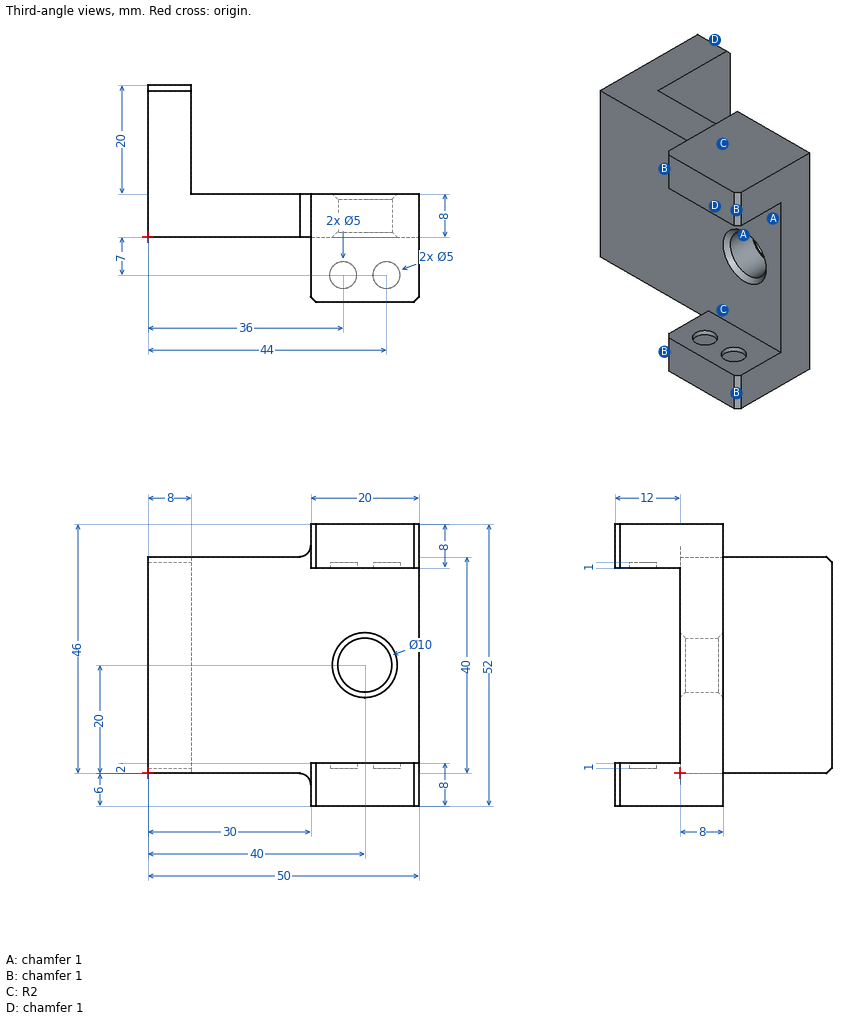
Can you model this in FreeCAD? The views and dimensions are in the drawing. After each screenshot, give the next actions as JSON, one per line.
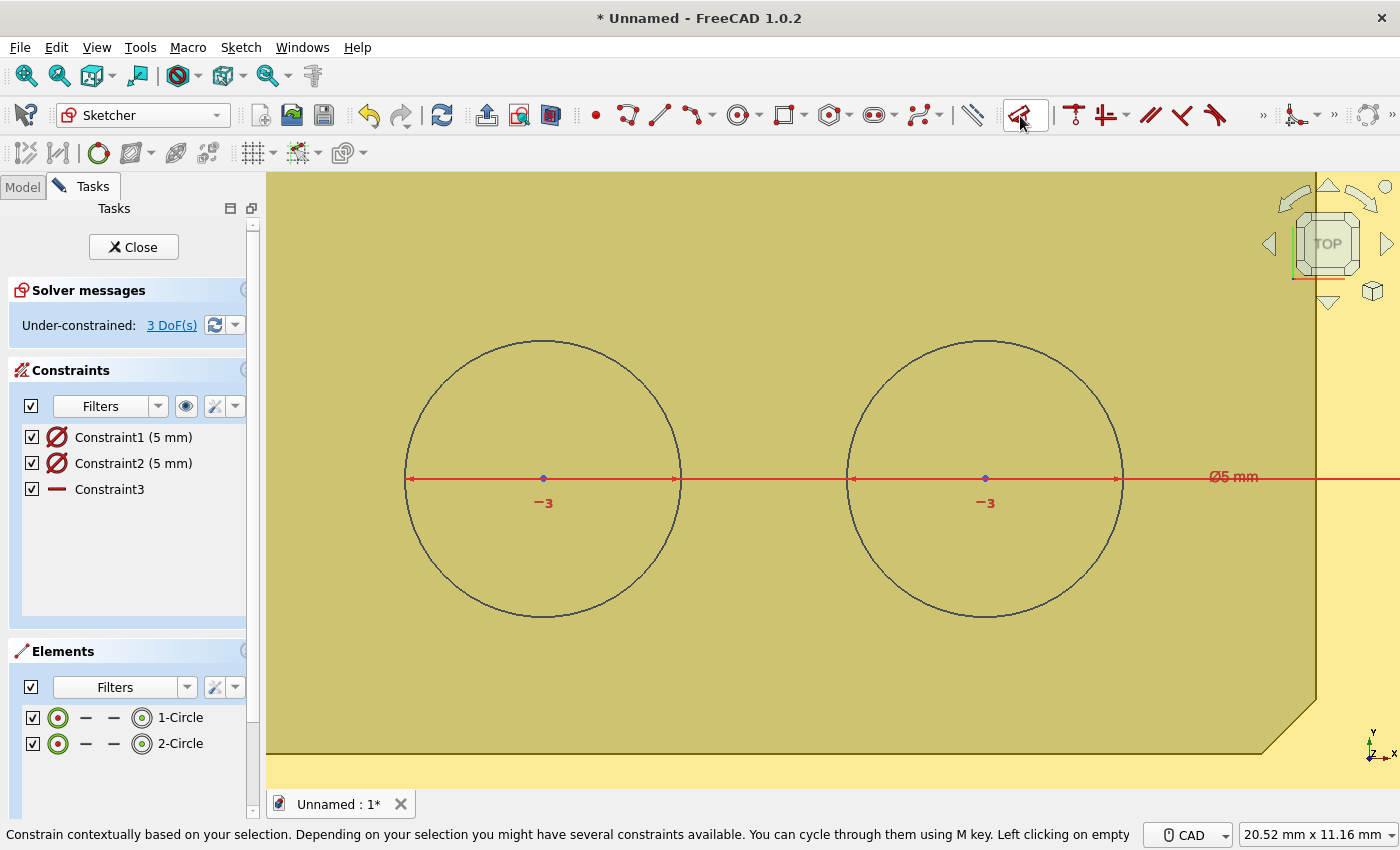
{"action": "left_click", "coordinate": [985, 479]}
{"action": "left_click", "coordinate": [1019, 275]}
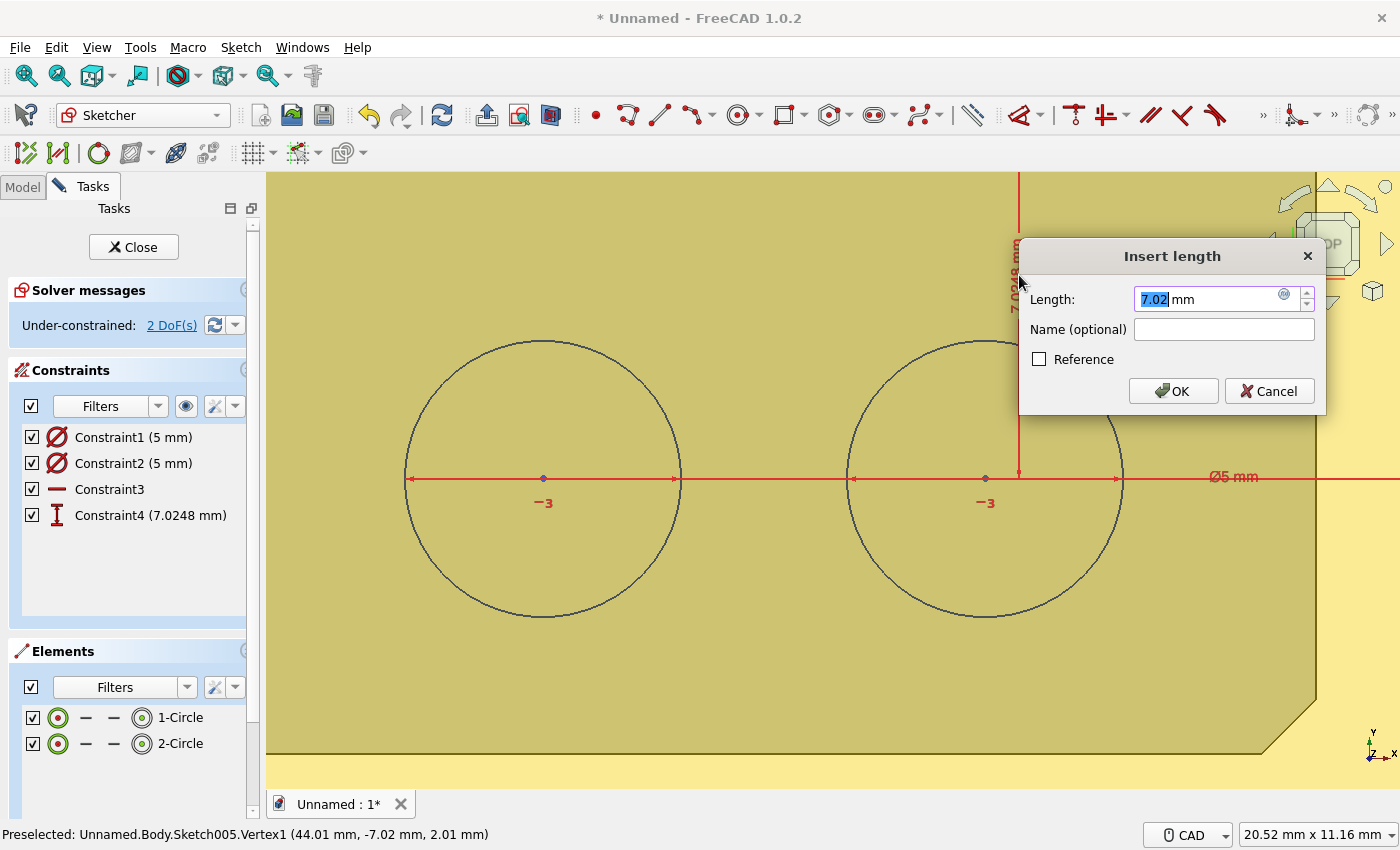
{"action": "type", "text": "7"}
{"action": "key", "text": "Return"}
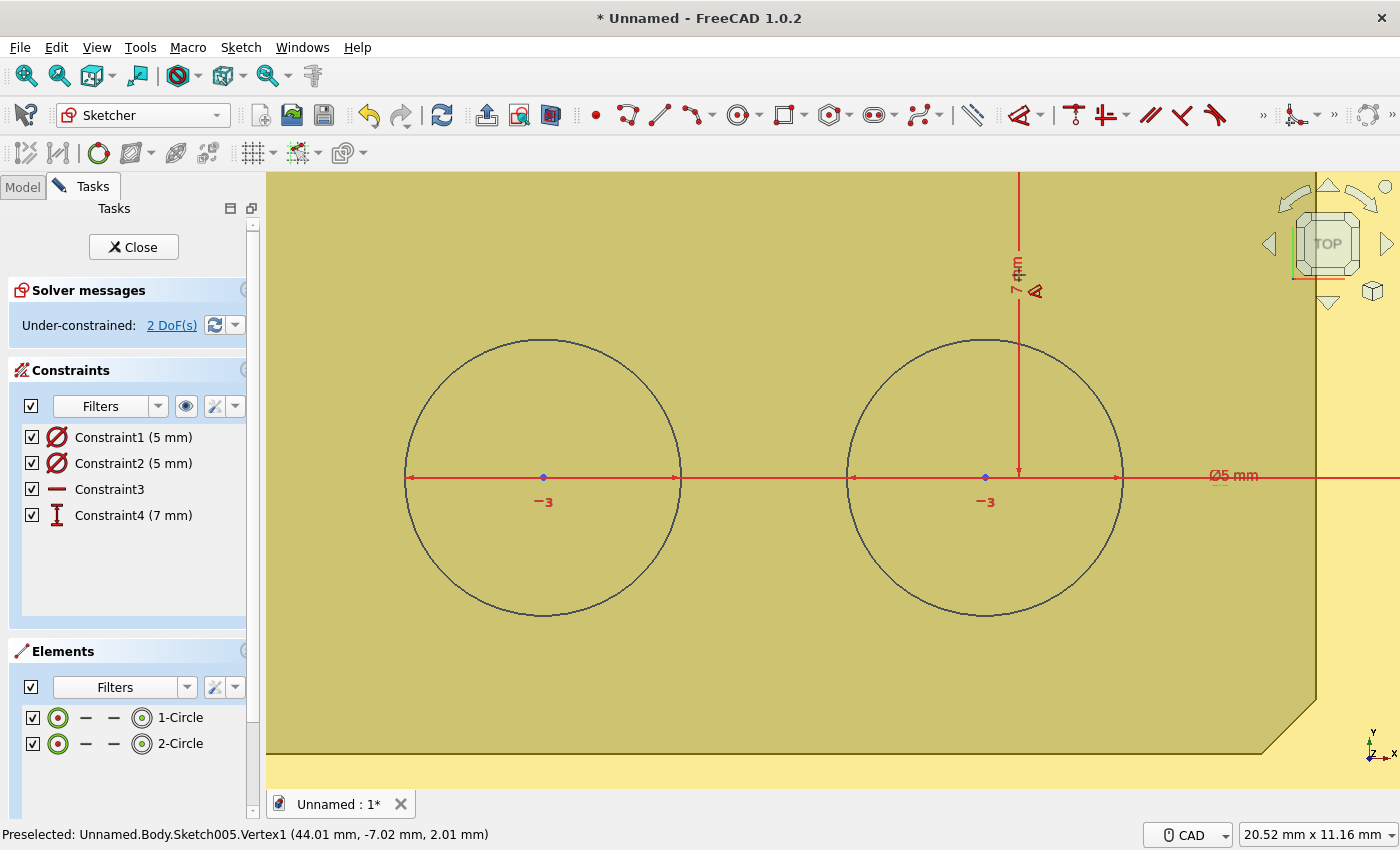
{"action": "left_click", "coordinate": [985, 478]}
{"action": "left_click", "coordinate": [640, 512]}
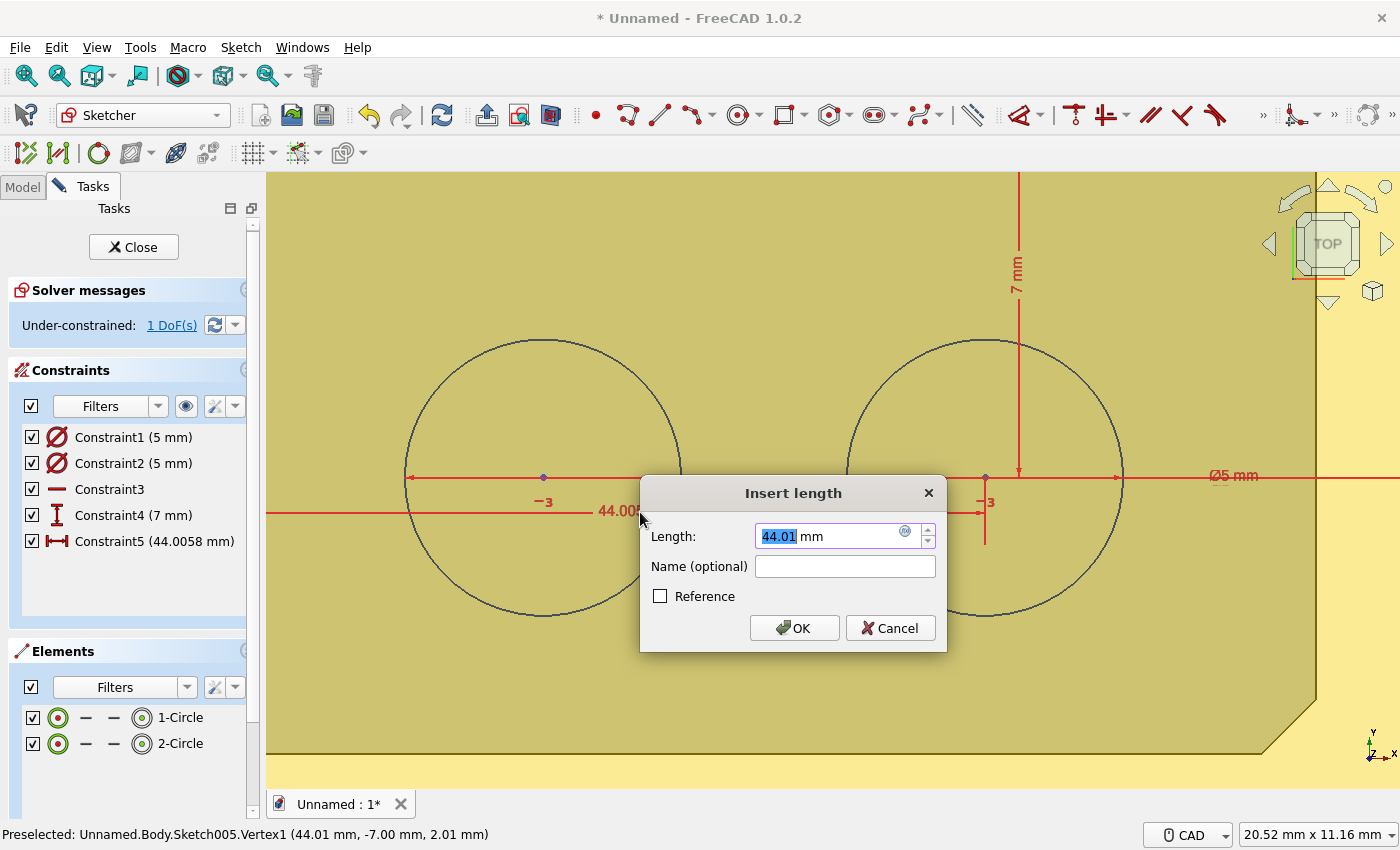
{"action": "type", "text": "44"}
{"action": "key", "text": "Return"}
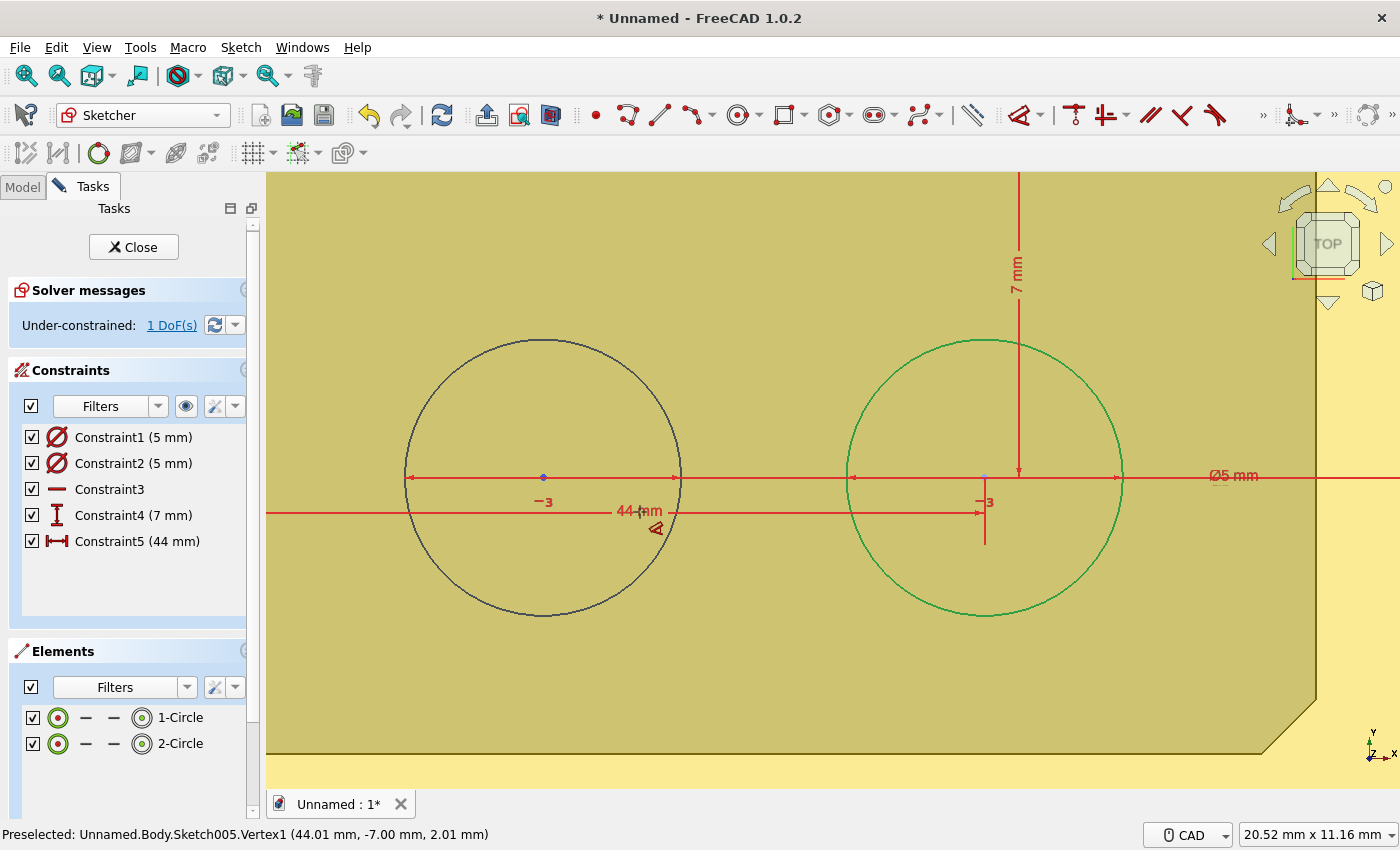
{"action": "left_click", "coordinate": [543, 478]}
{"action": "left_click", "coordinate": [361, 512]}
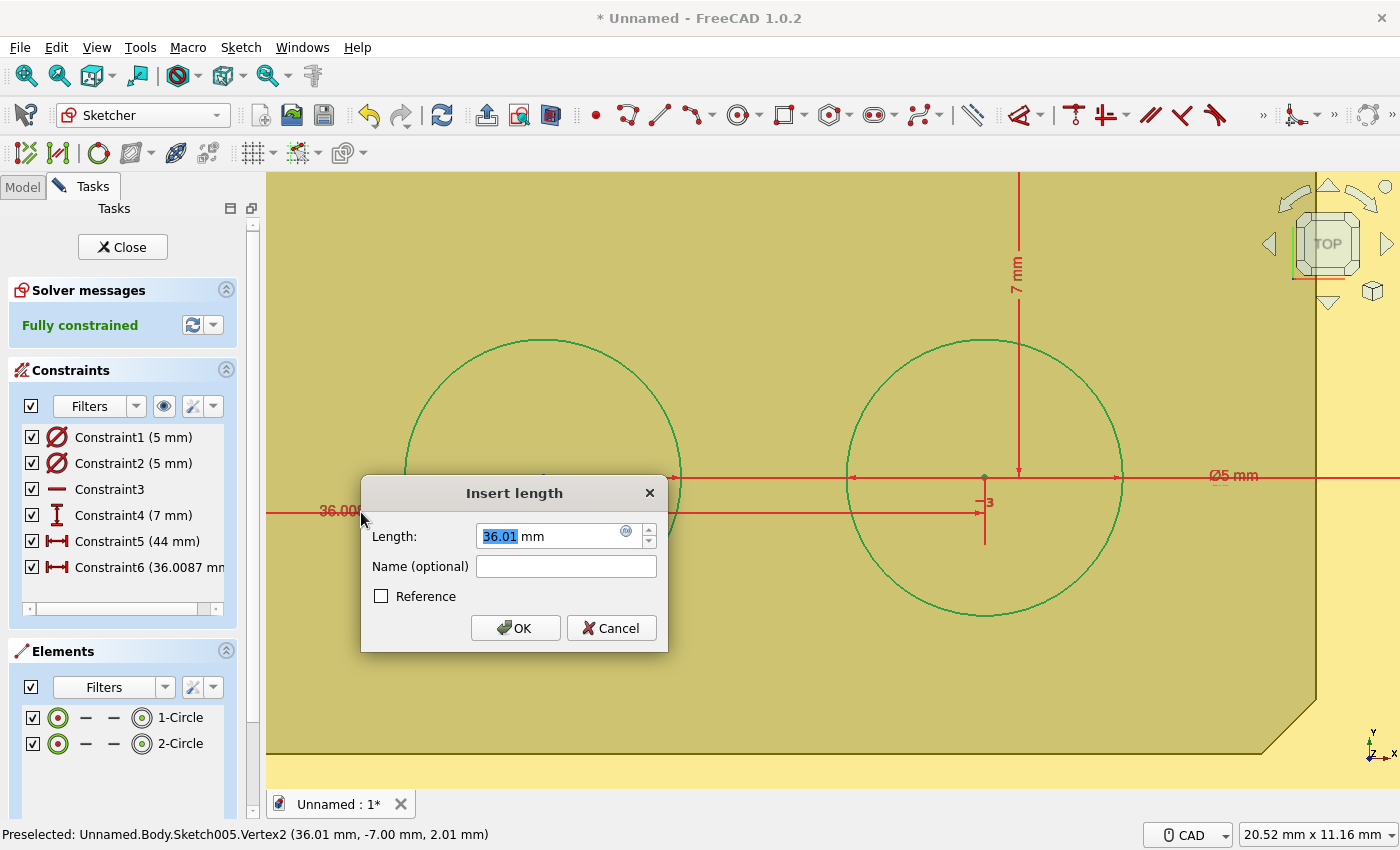
{"action": "type", "text": "36"}
{"action": "key", "text": "Return"}
{"action": "key", "text": "Escape"}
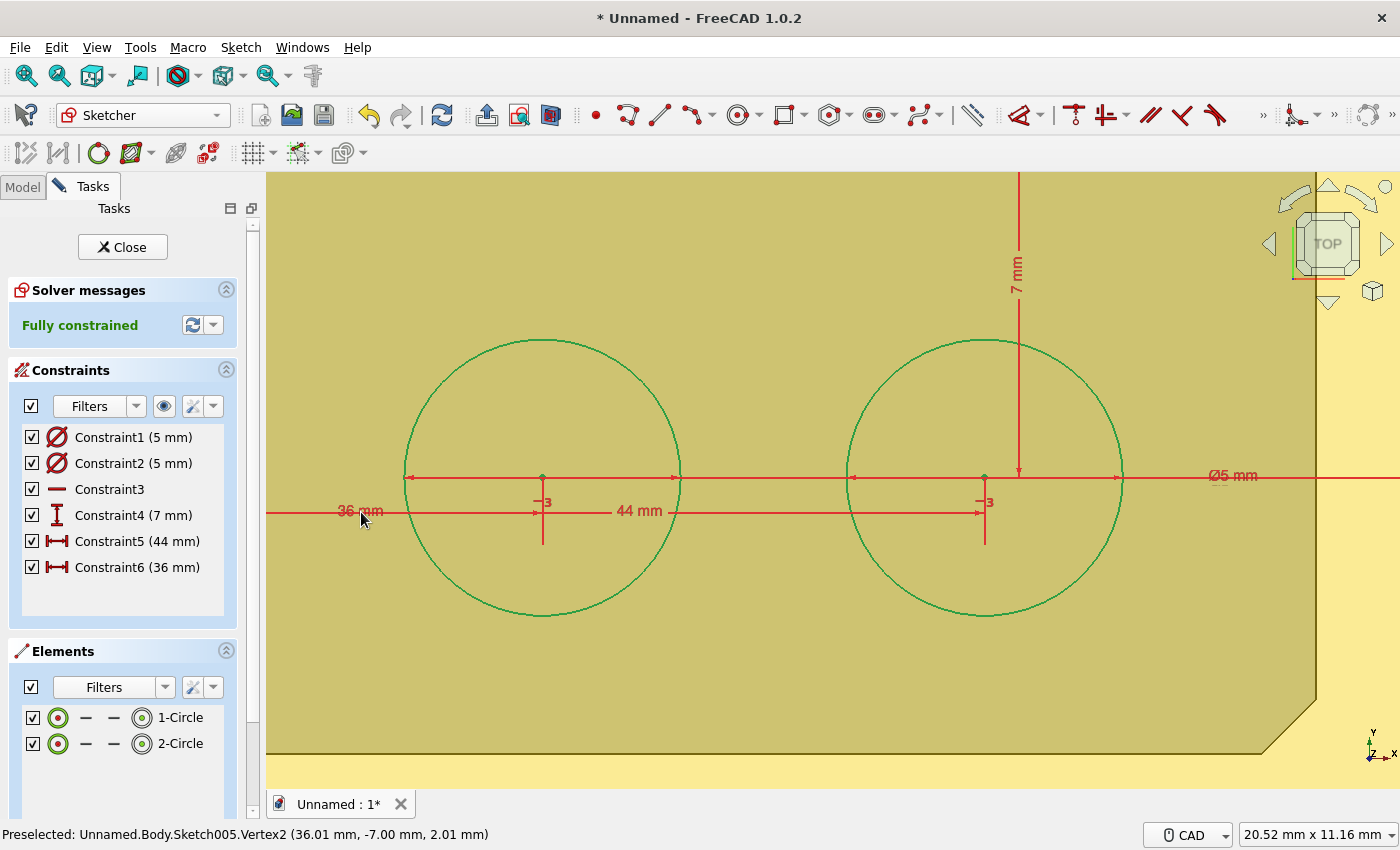
{"action": "left_click", "coordinate": [123, 247]}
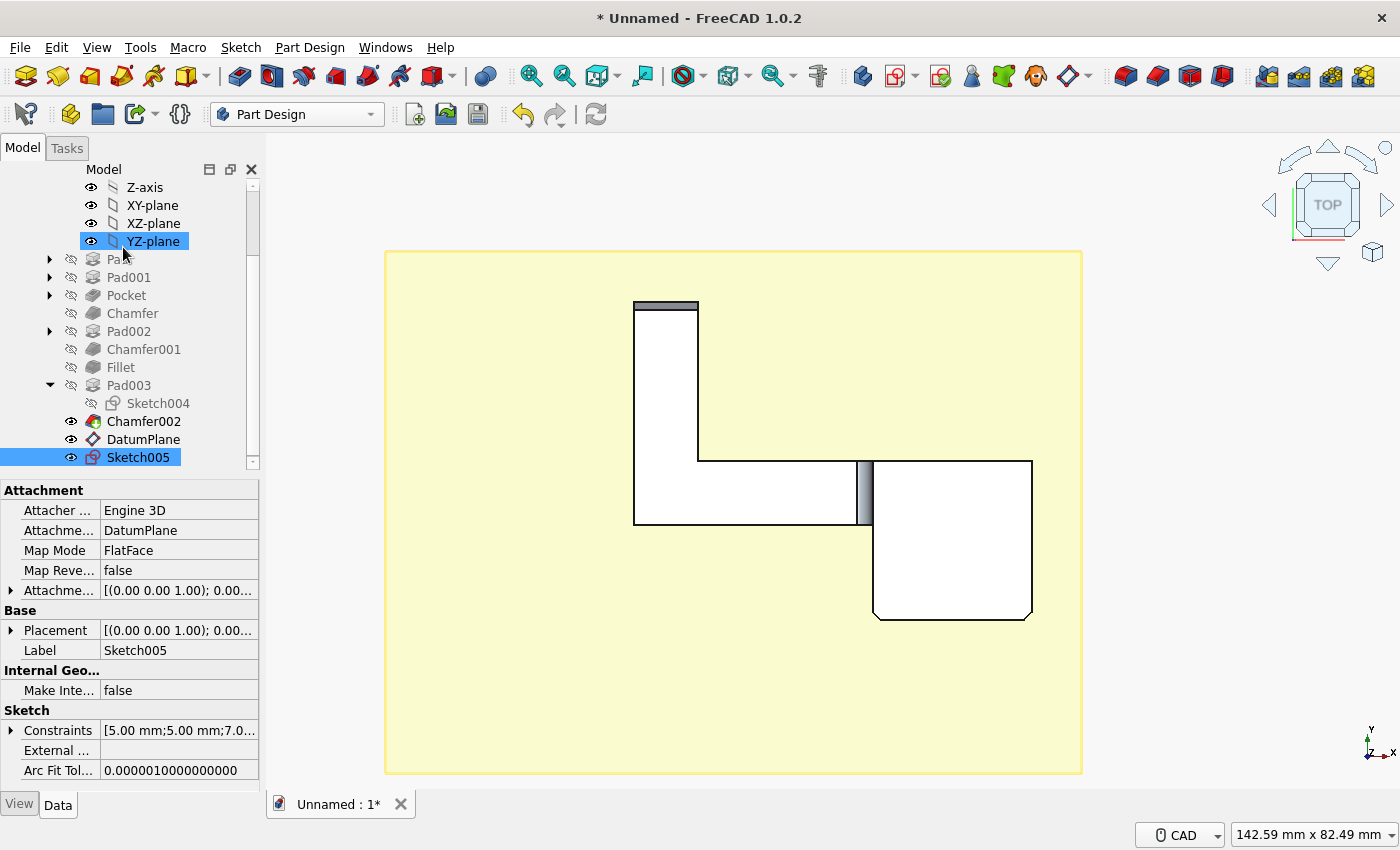
{"action": "left_click", "coordinate": [240, 76]}